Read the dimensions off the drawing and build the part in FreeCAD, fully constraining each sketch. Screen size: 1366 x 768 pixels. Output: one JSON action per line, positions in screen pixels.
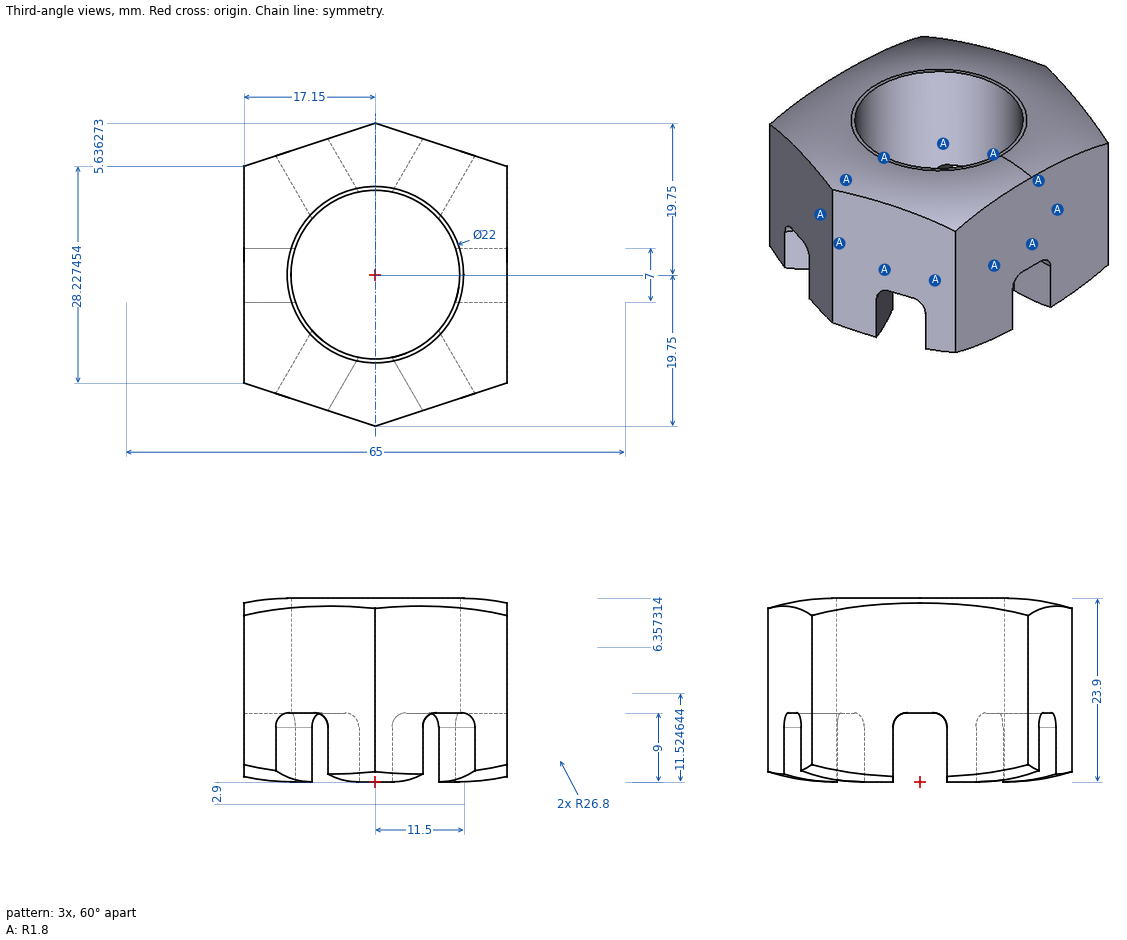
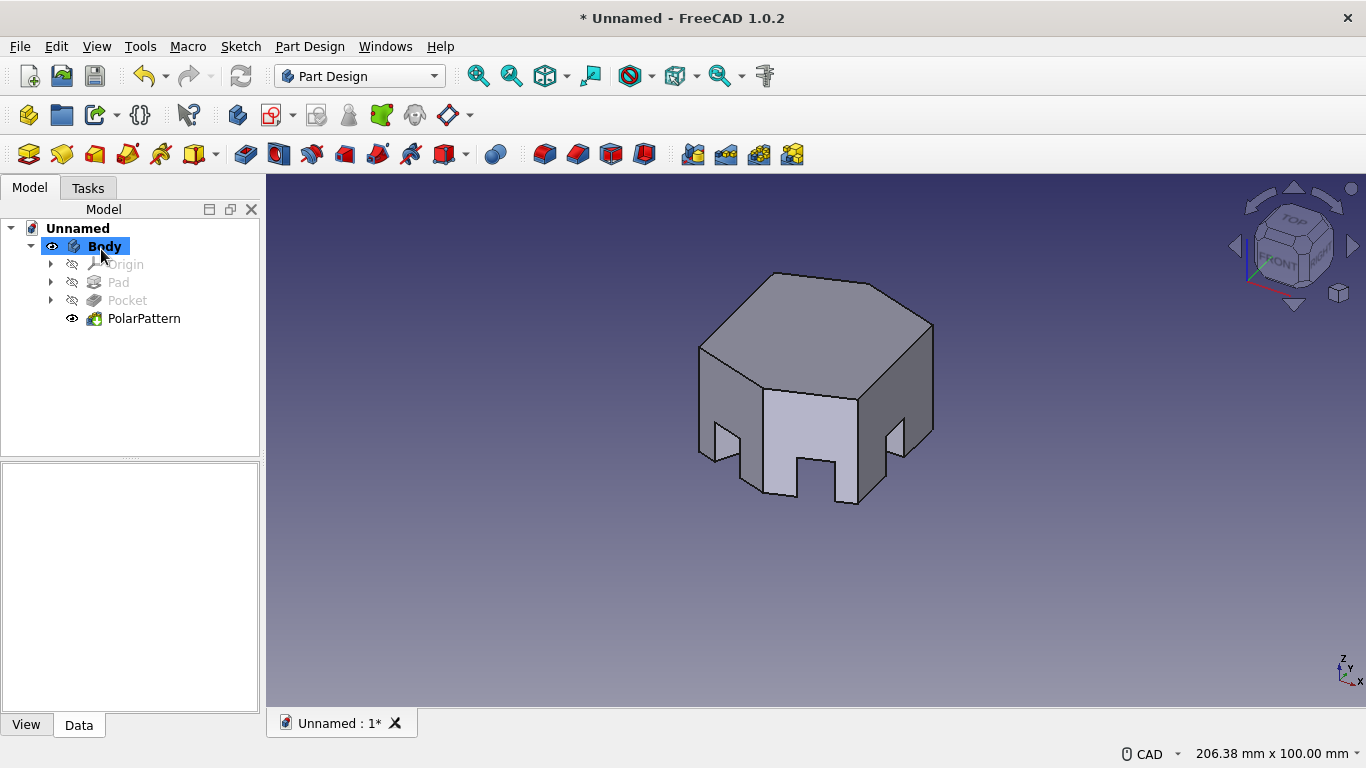
{"action": "left_click", "coordinate": [816, 335]}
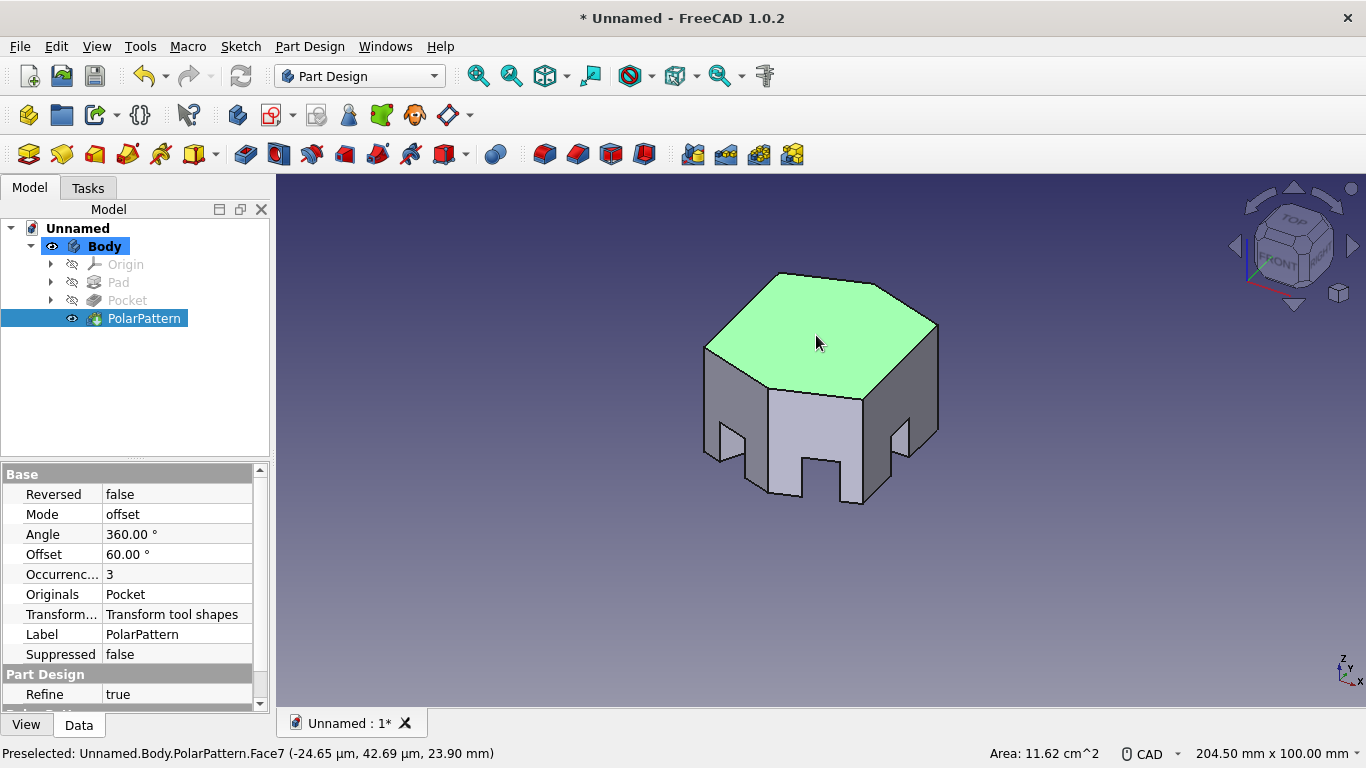
{"action": "left_click", "coordinate": [270, 116]}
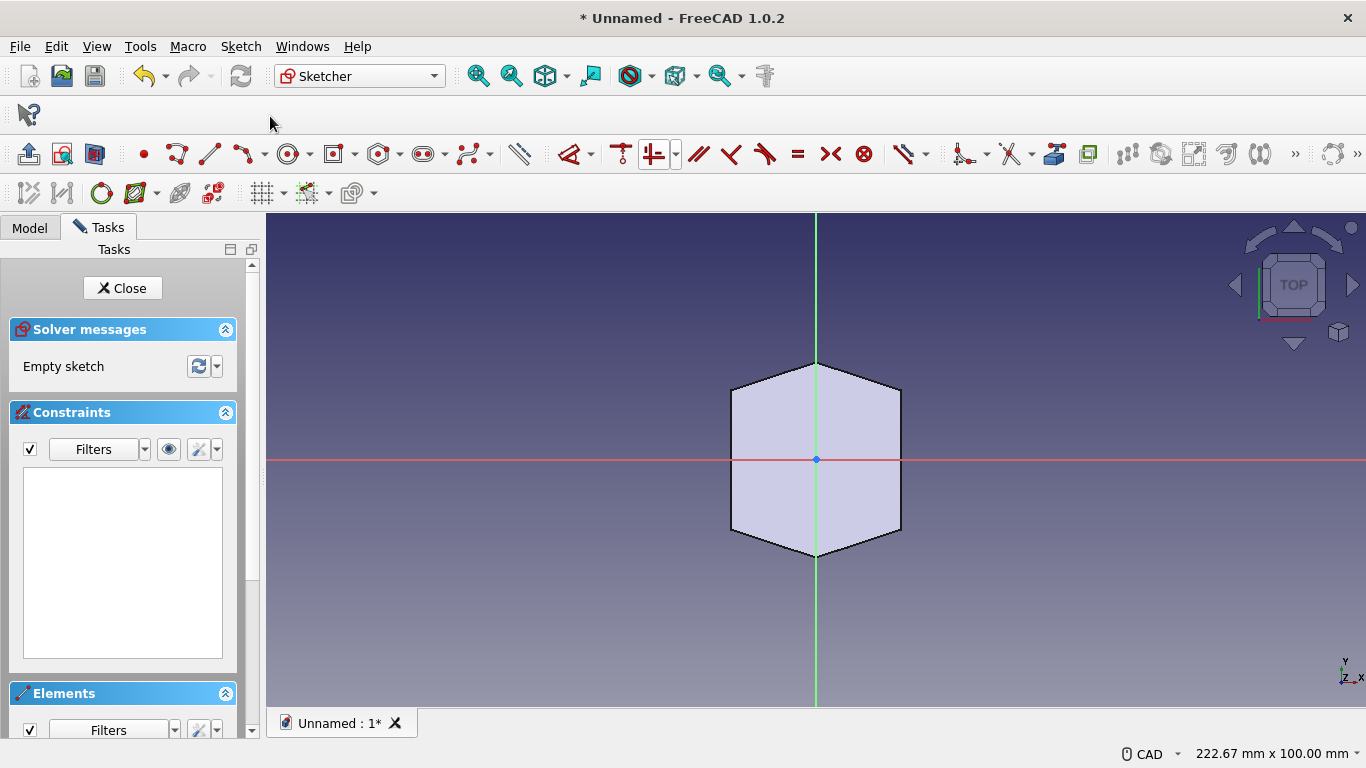
{"action": "scroll", "coordinate": [856, 460], "scroll_direction": "up", "scroll_amount": 5}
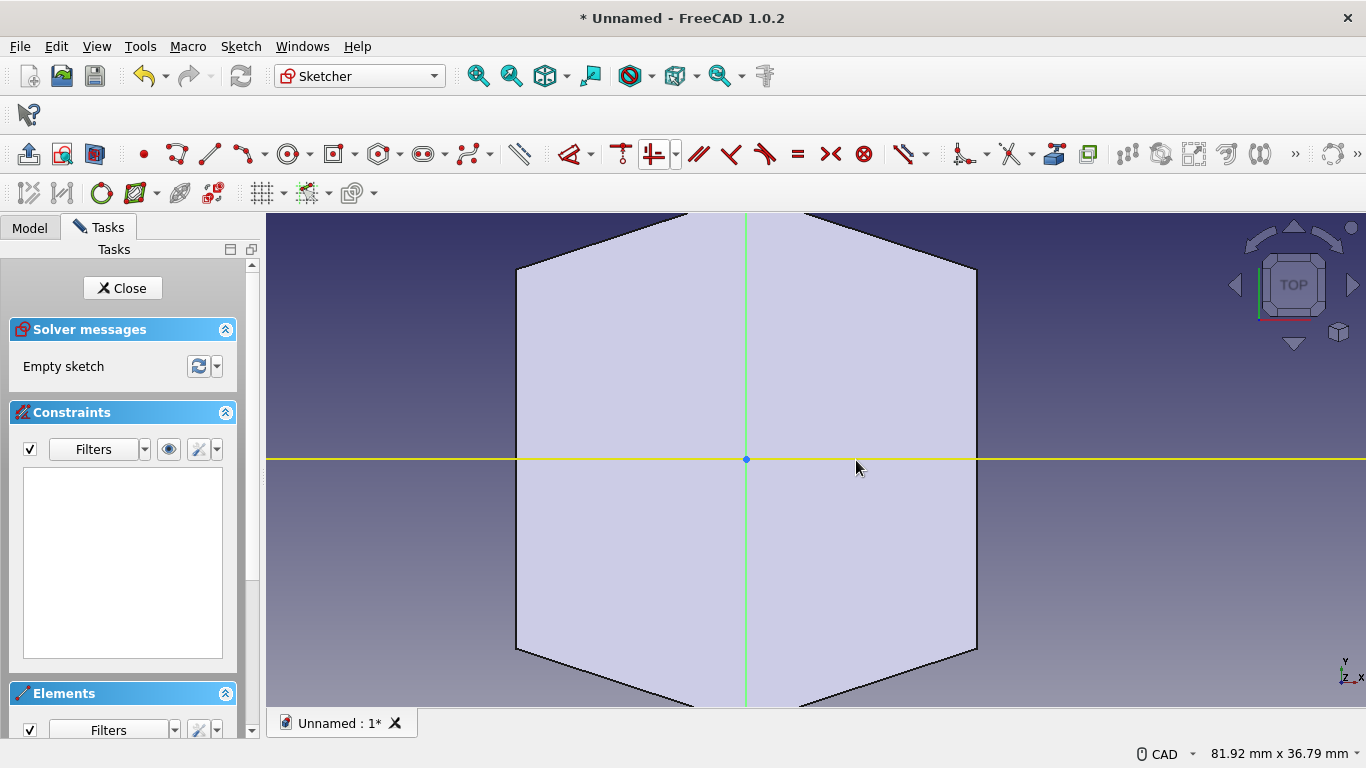
{"action": "left_click", "coordinate": [288, 154]}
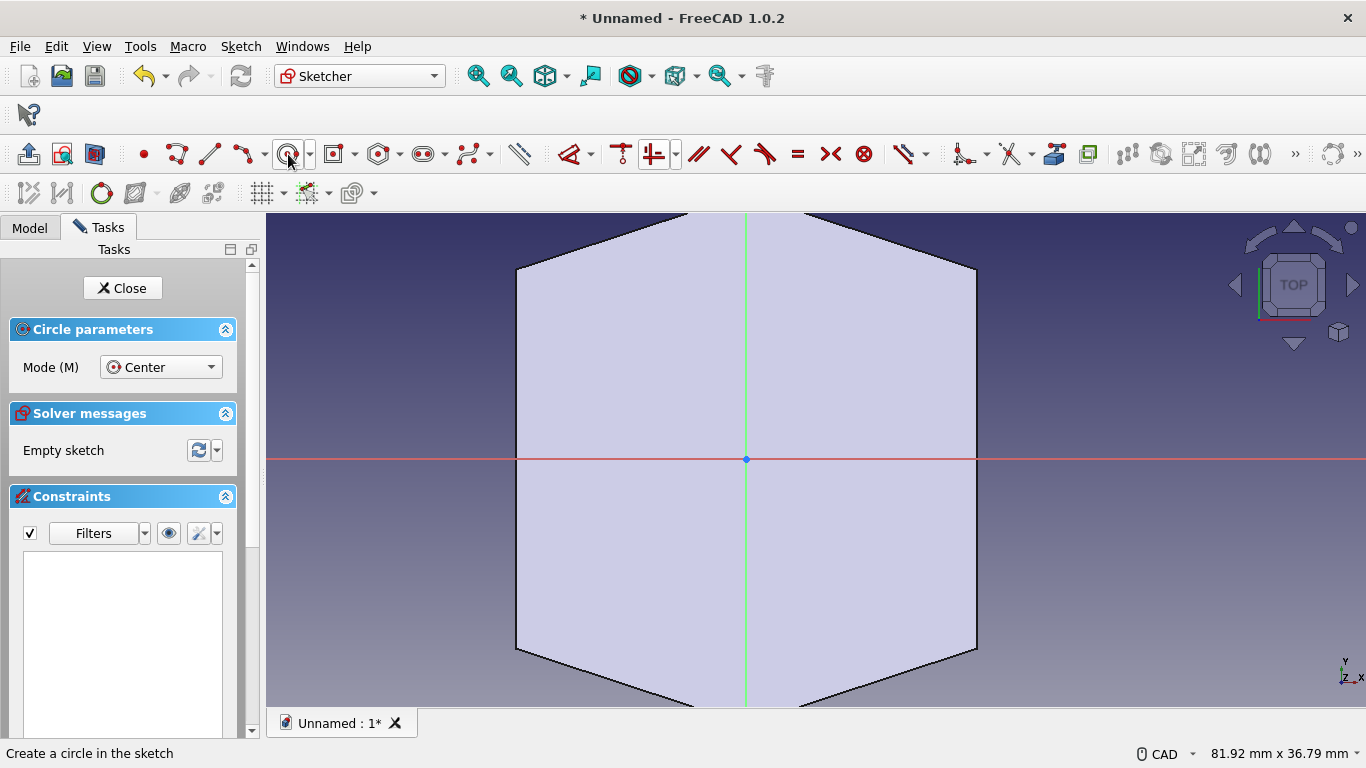
{"action": "left_click", "coordinate": [746, 459]}
{"action": "mouse_move", "coordinate": [851, 355]}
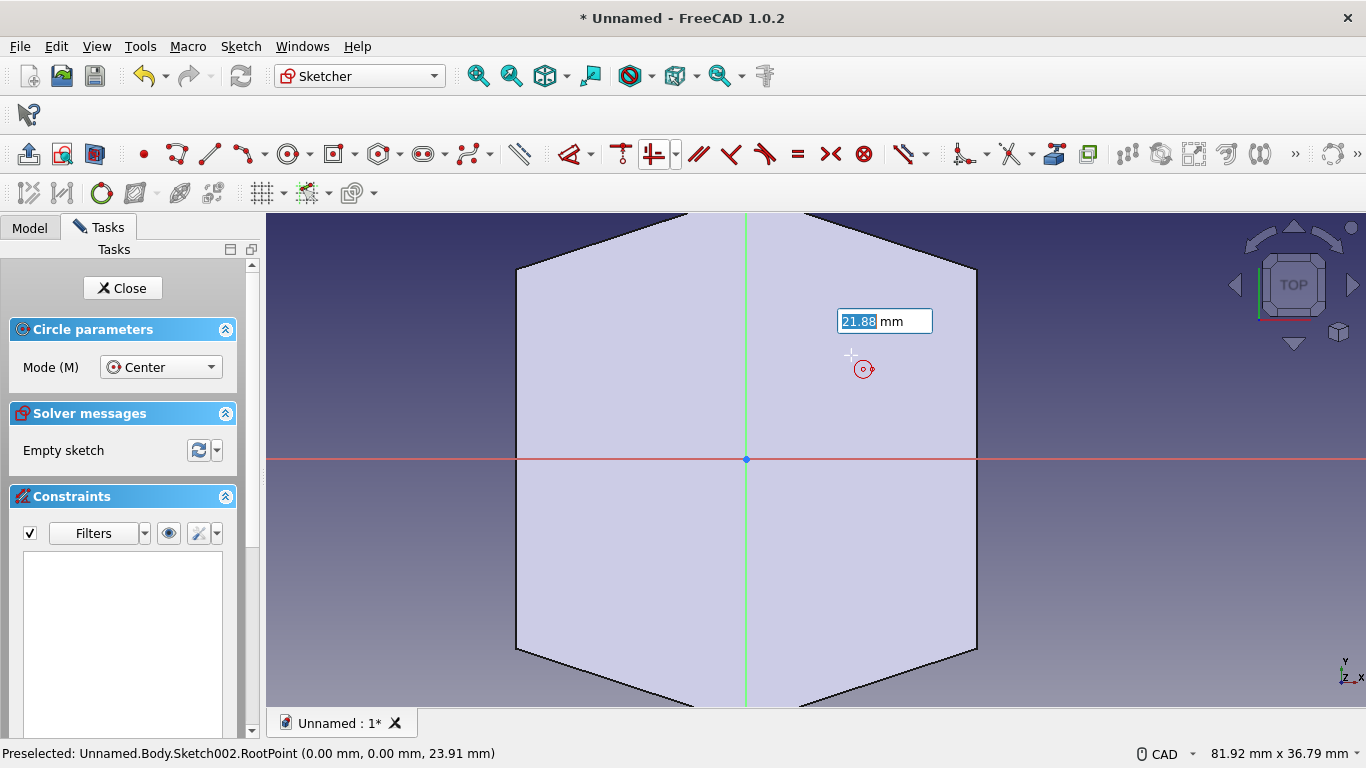
{"action": "type", "text": "22"}
{"action": "key", "text": "Return"}
{"action": "key", "text": "Escape"}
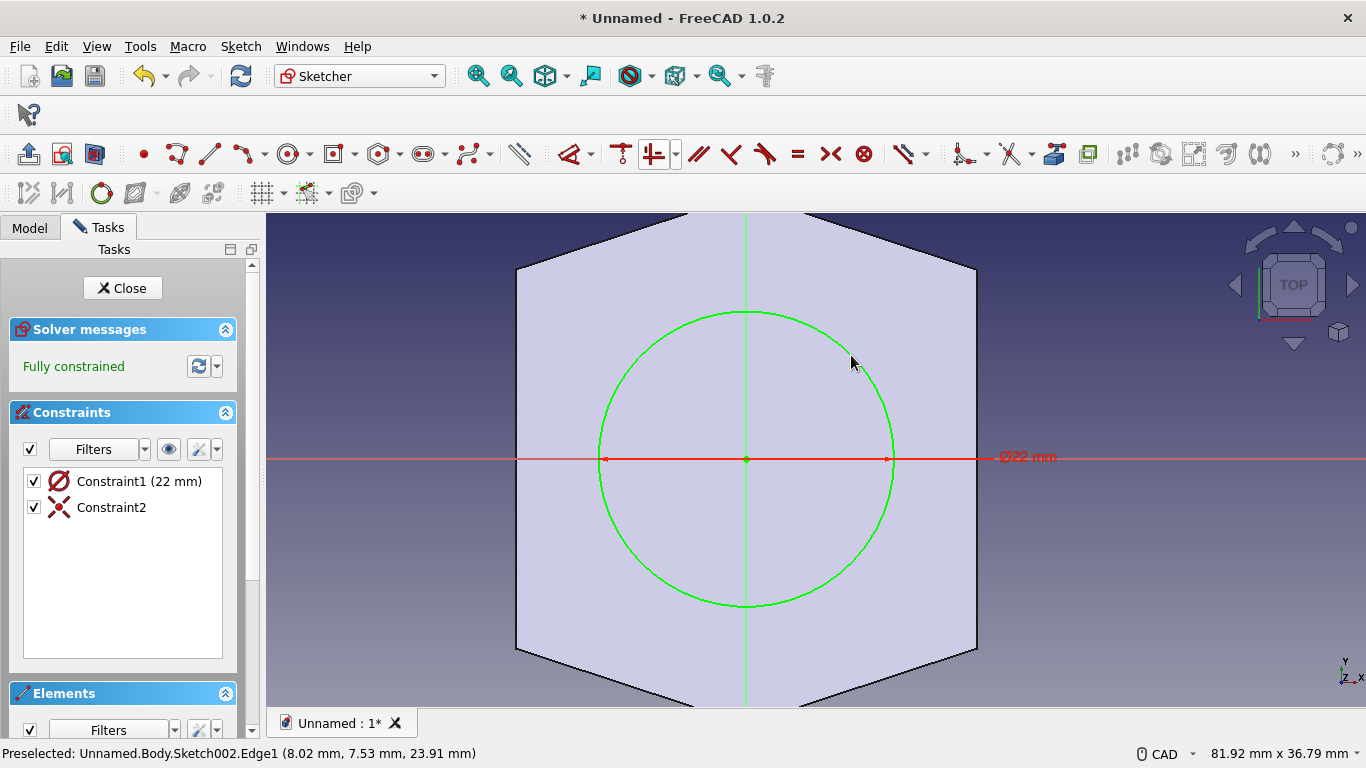
{"action": "left_click", "coordinate": [123, 288]}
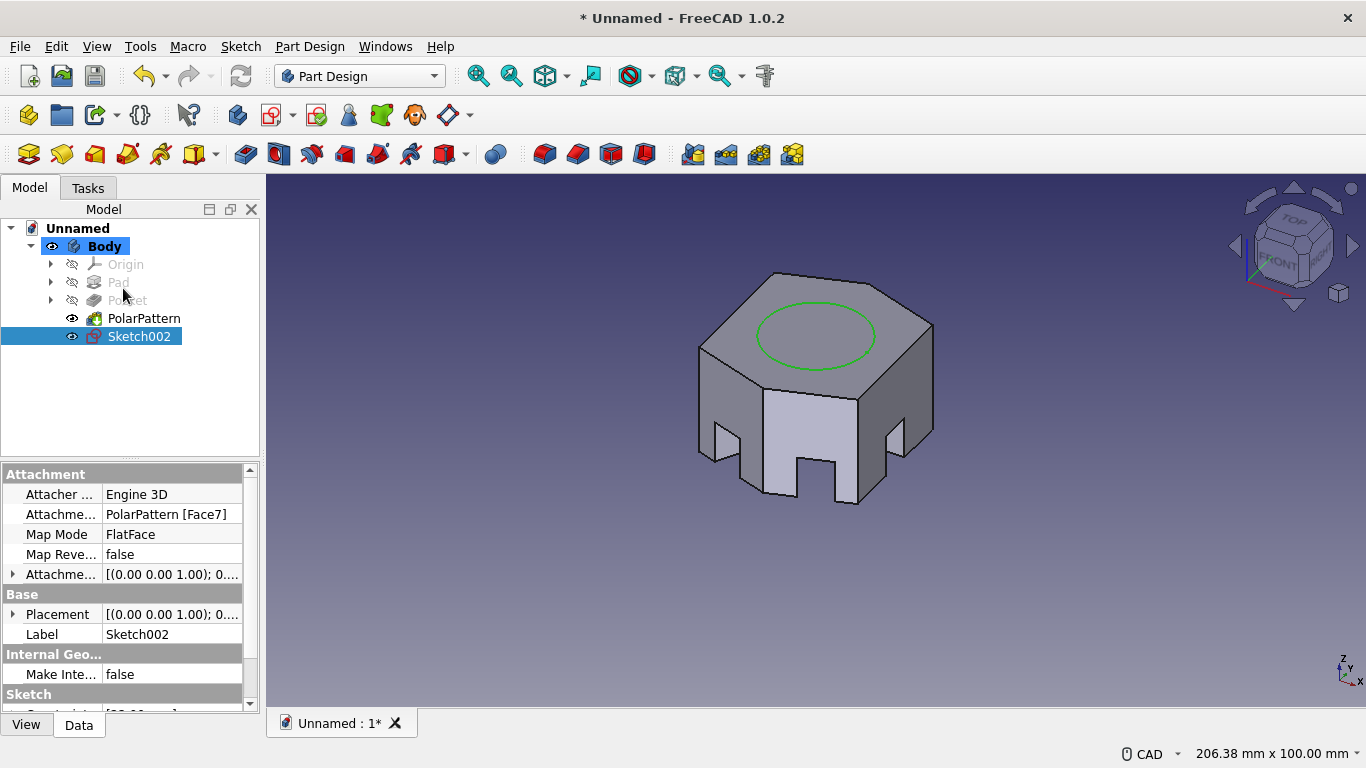
{"action": "left_click", "coordinate": [246, 154]}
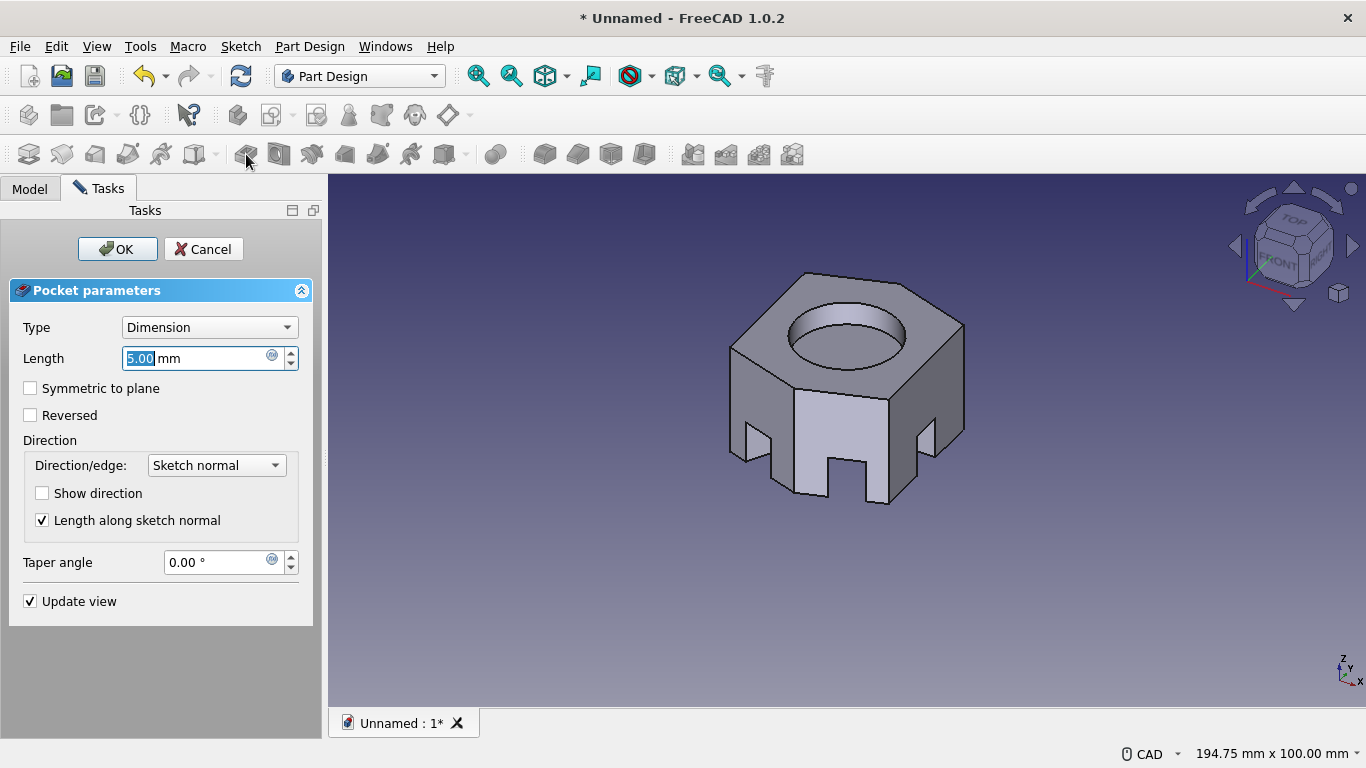
{"action": "left_click", "coordinate": [210, 328]}